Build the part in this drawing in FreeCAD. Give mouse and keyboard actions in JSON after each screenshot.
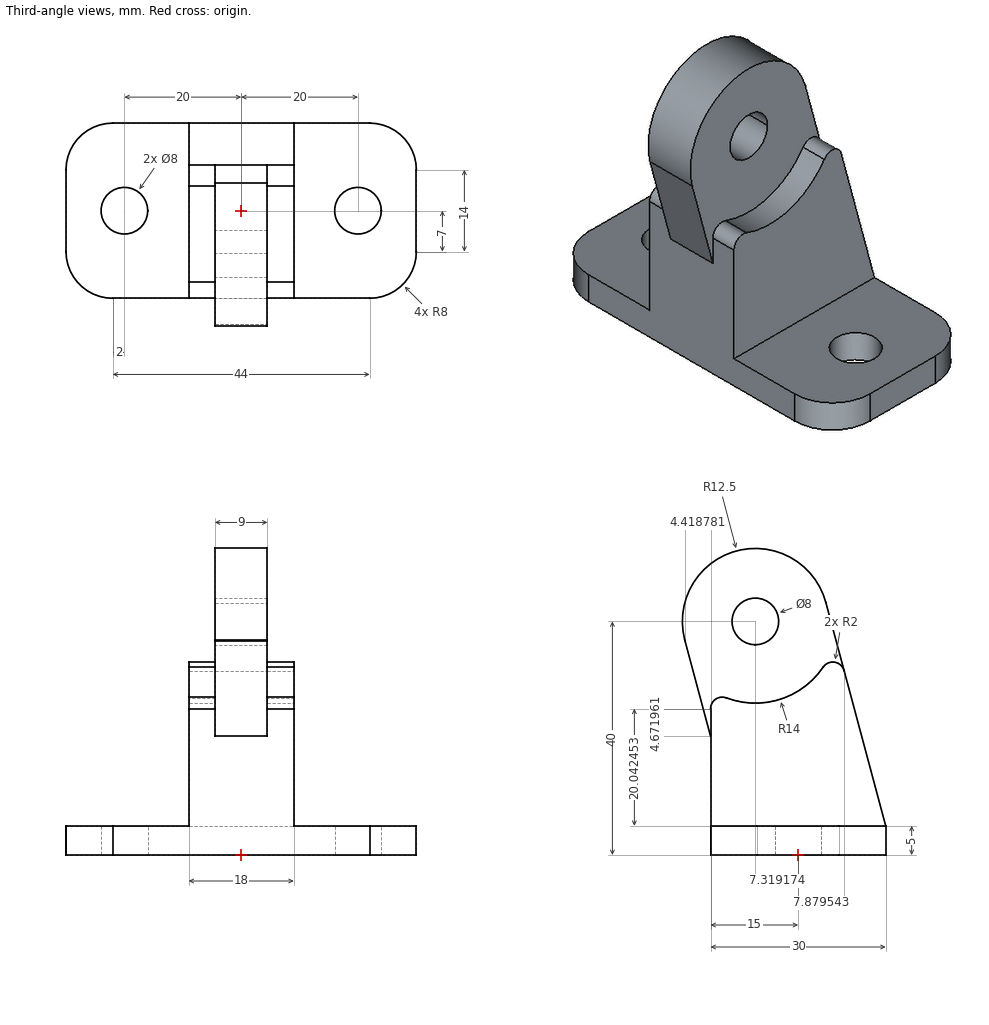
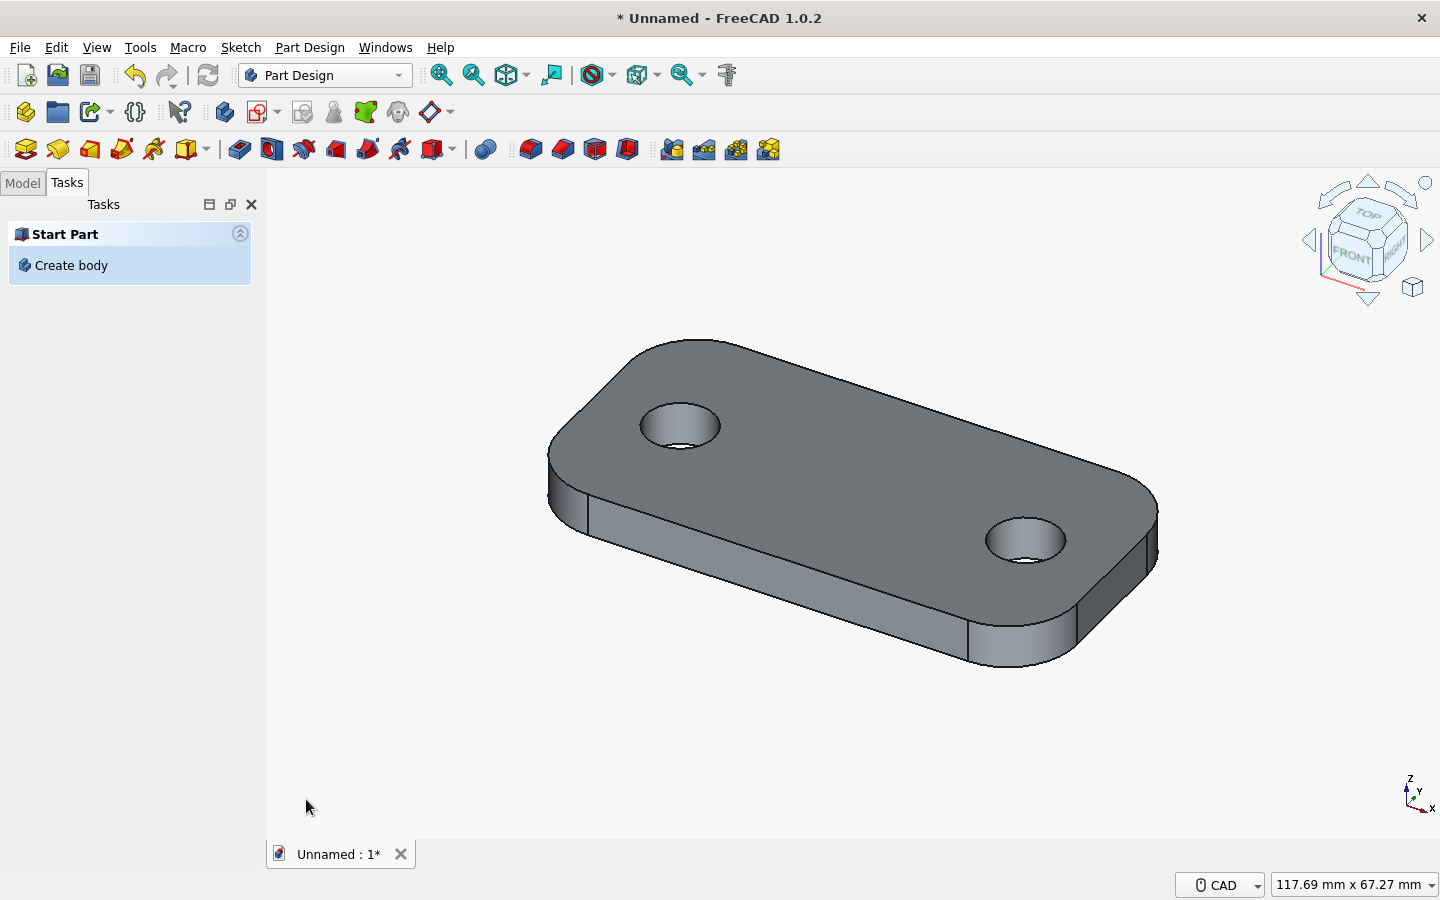
{"action": "left_click", "coordinate": [258, 112]}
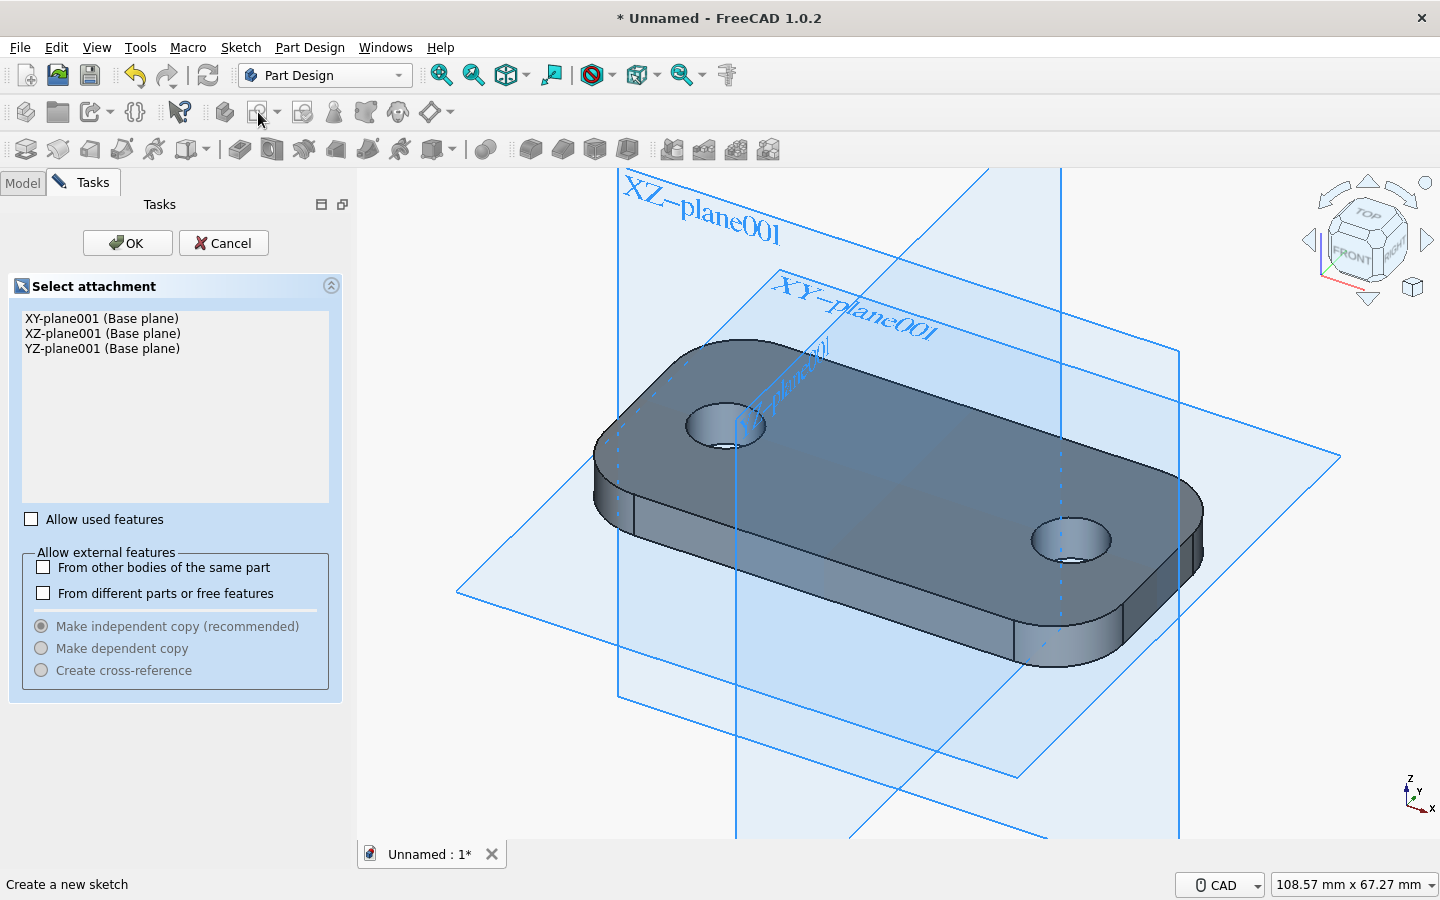
{"action": "left_click", "coordinate": [82, 348]}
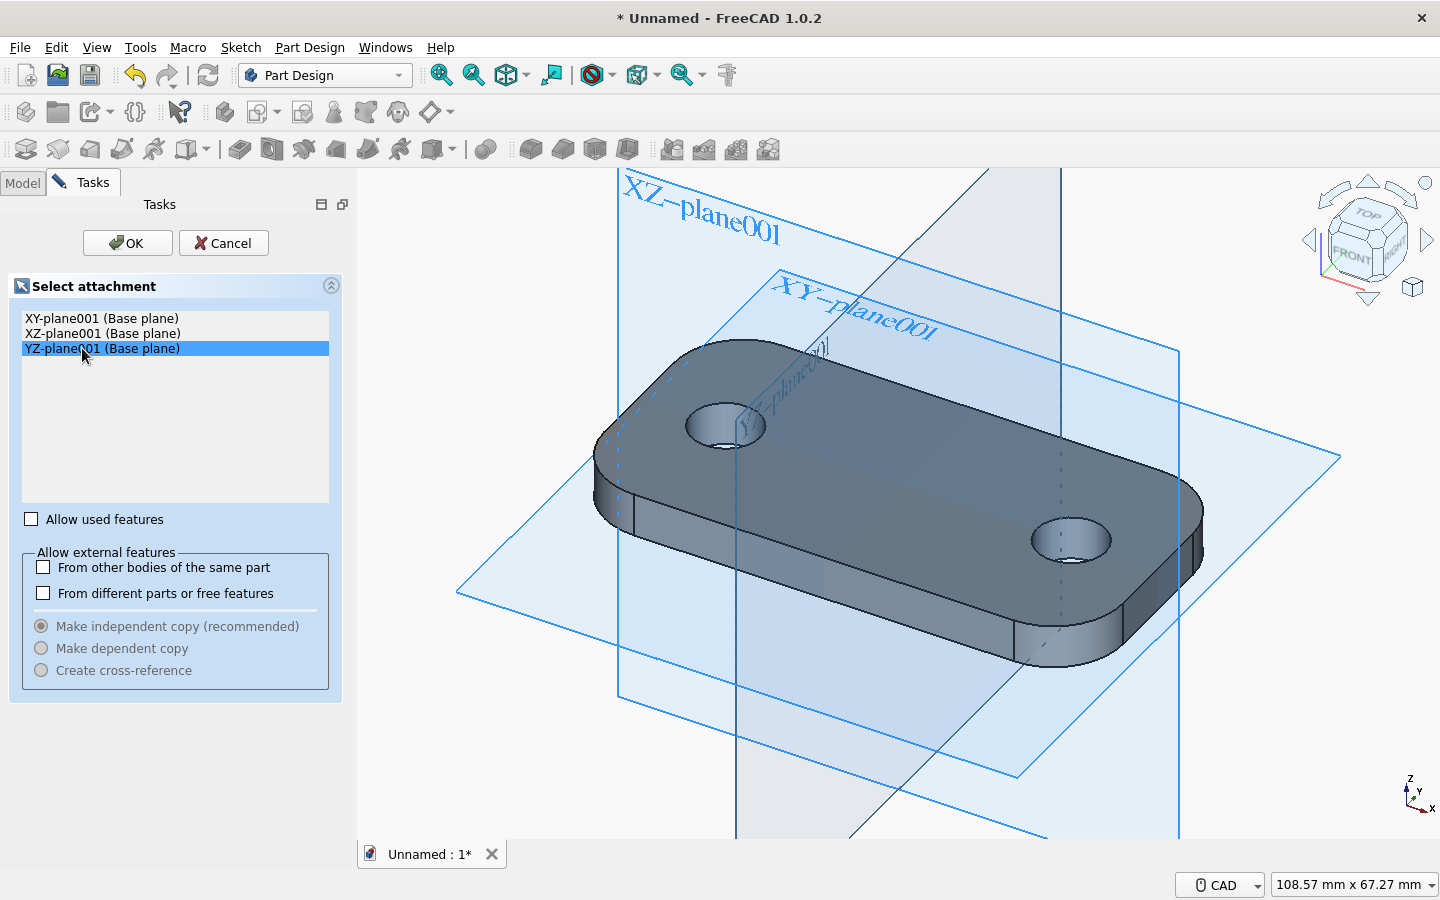
{"action": "left_click", "coordinate": [128, 243]}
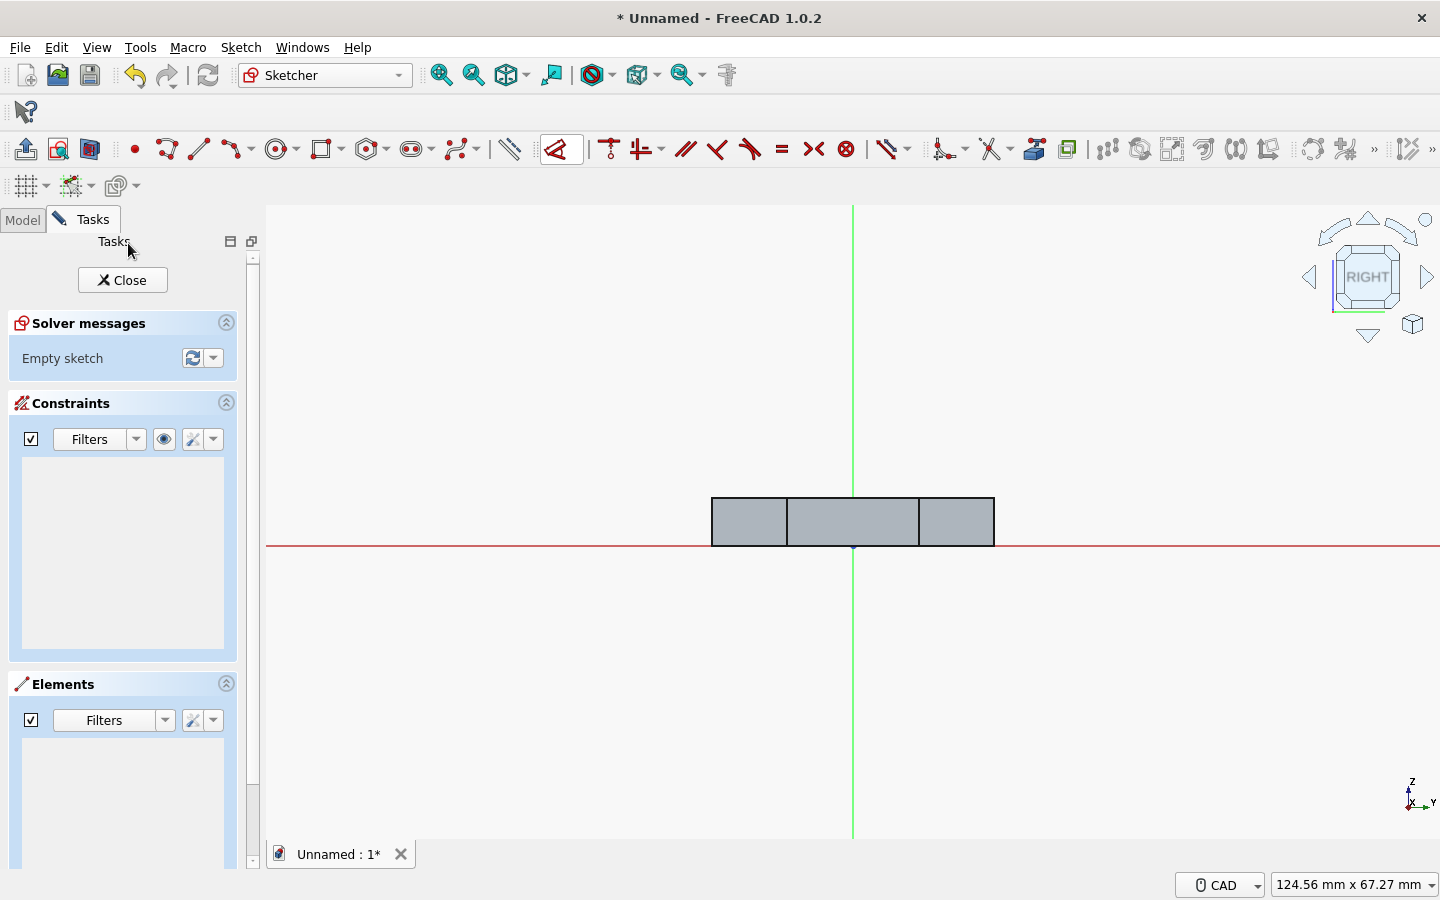
{"action": "scroll", "coordinate": [756, 811], "scroll_direction": "down", "scroll_amount": 2}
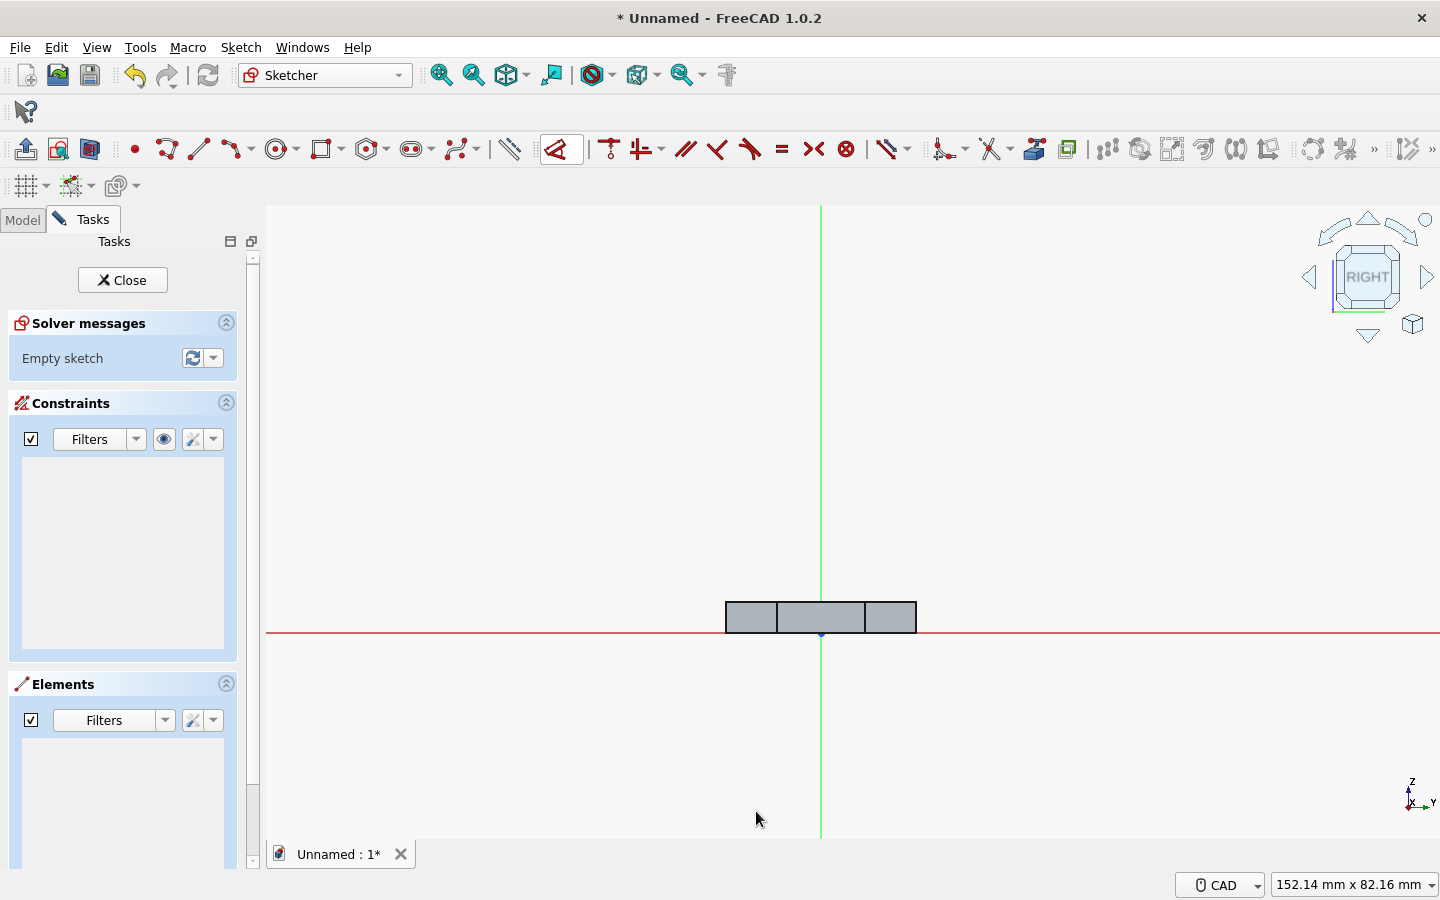
{"action": "key", "text": "g l"}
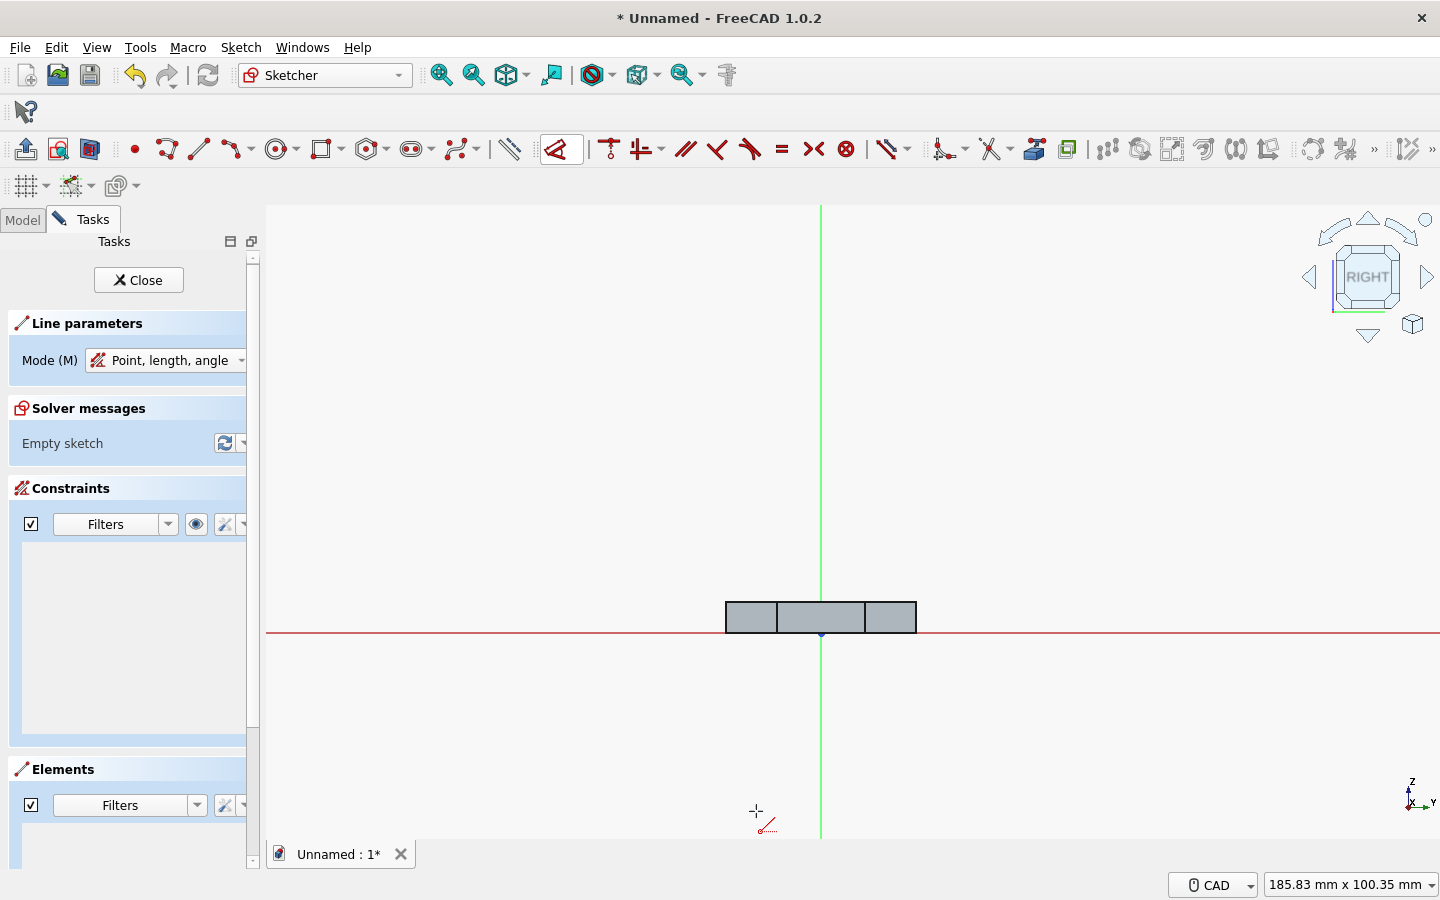
{"action": "left_click", "coordinate": [871, 434]}
{"action": "left_click", "coordinate": [851, 360]}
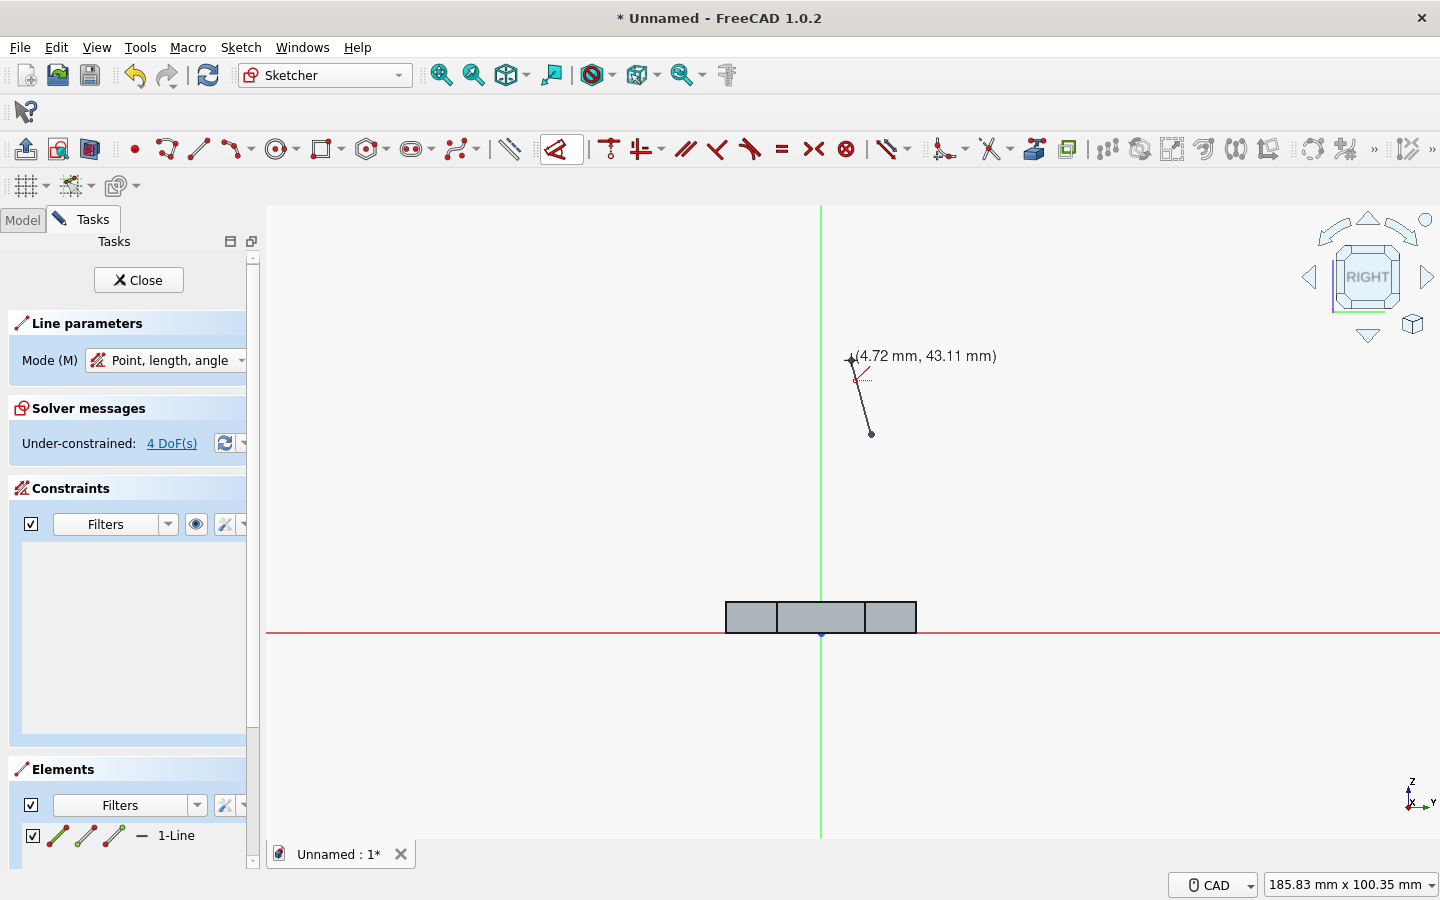
{"action": "key", "text": "g m"}